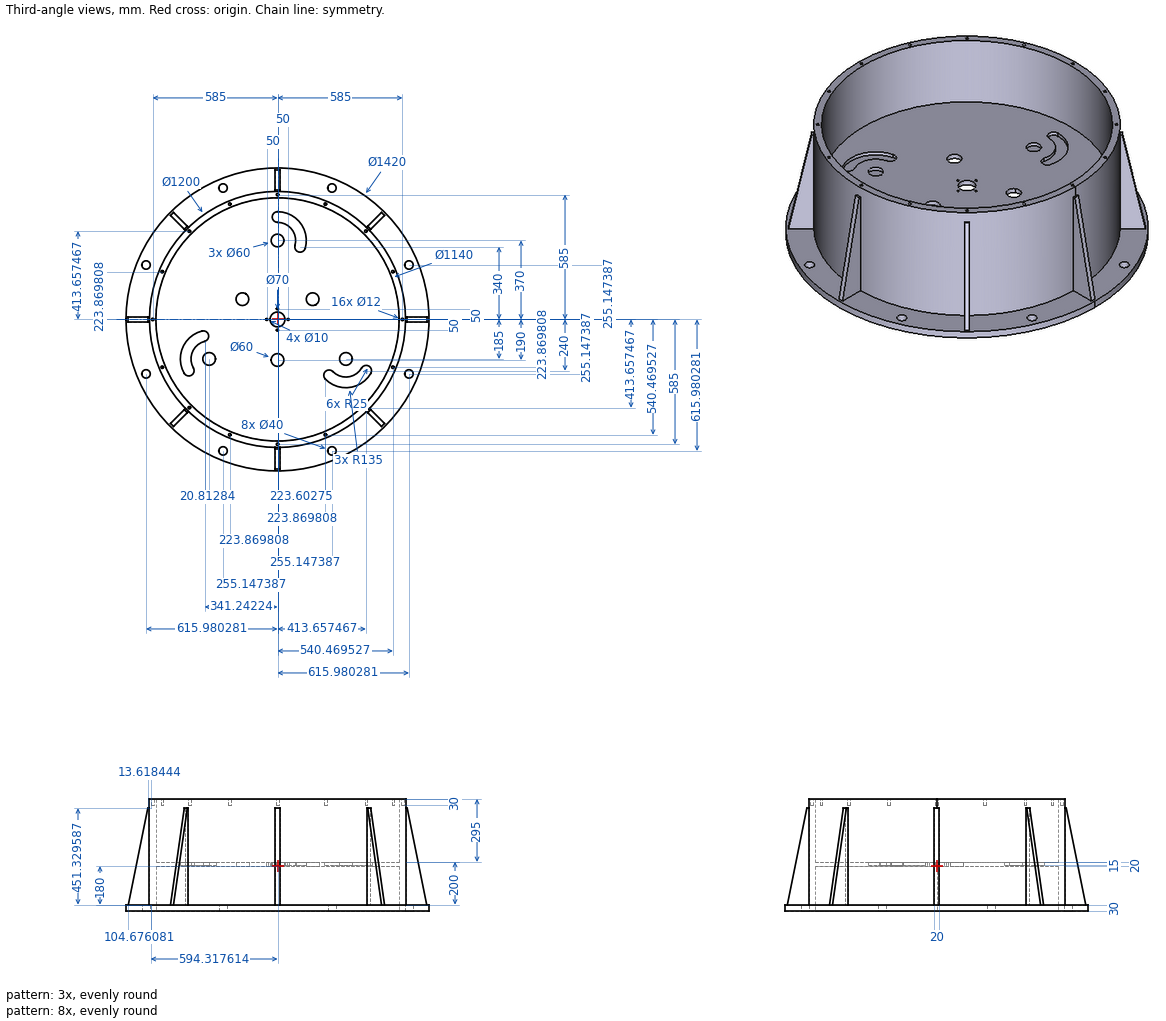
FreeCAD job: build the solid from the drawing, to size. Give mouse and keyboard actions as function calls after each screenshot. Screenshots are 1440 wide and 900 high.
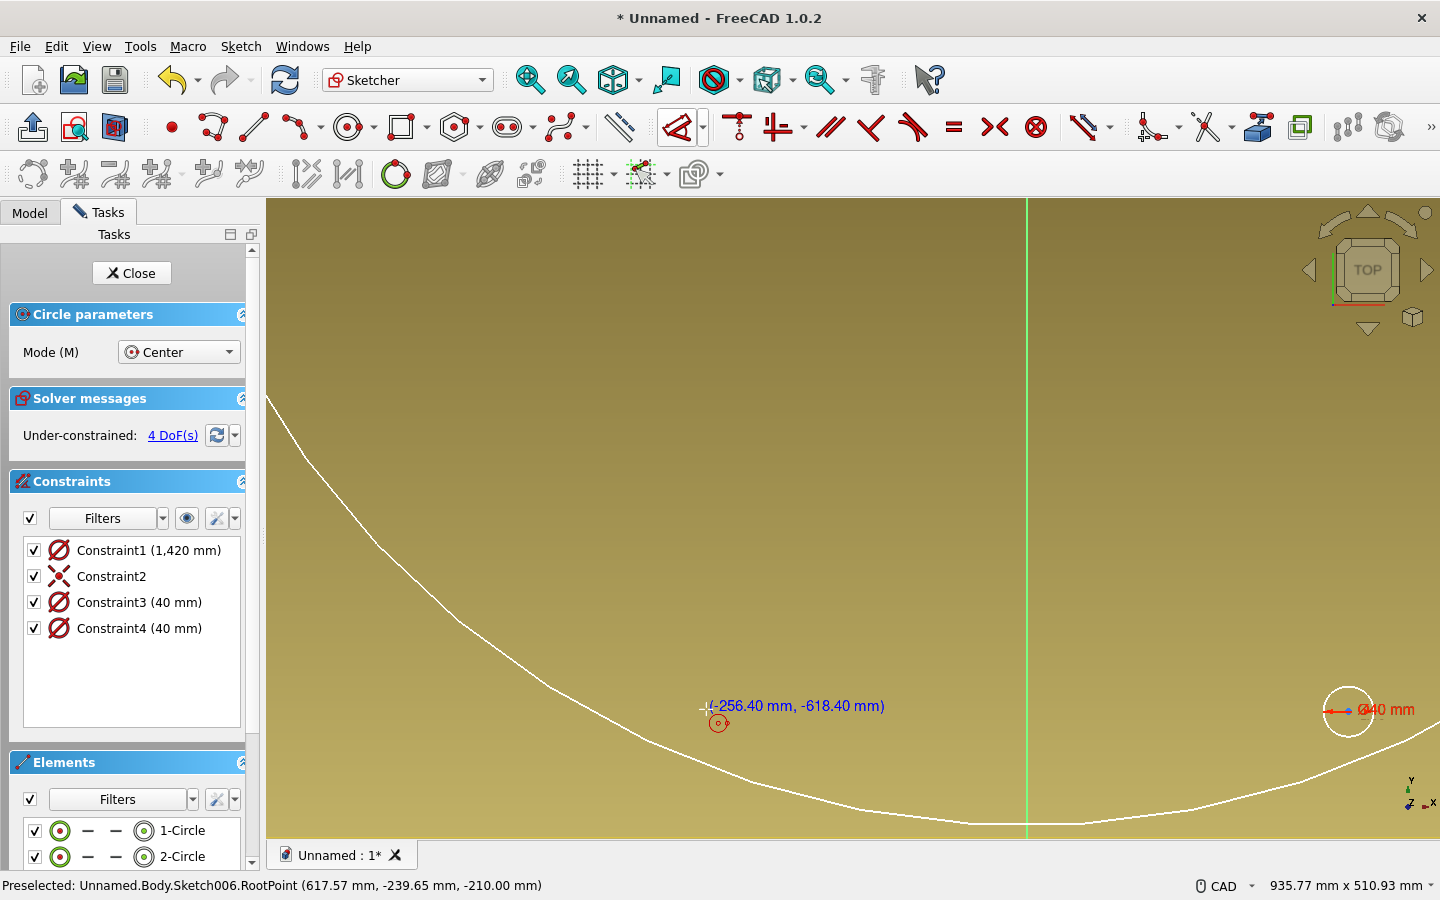
scroll(705, 710, down, 7)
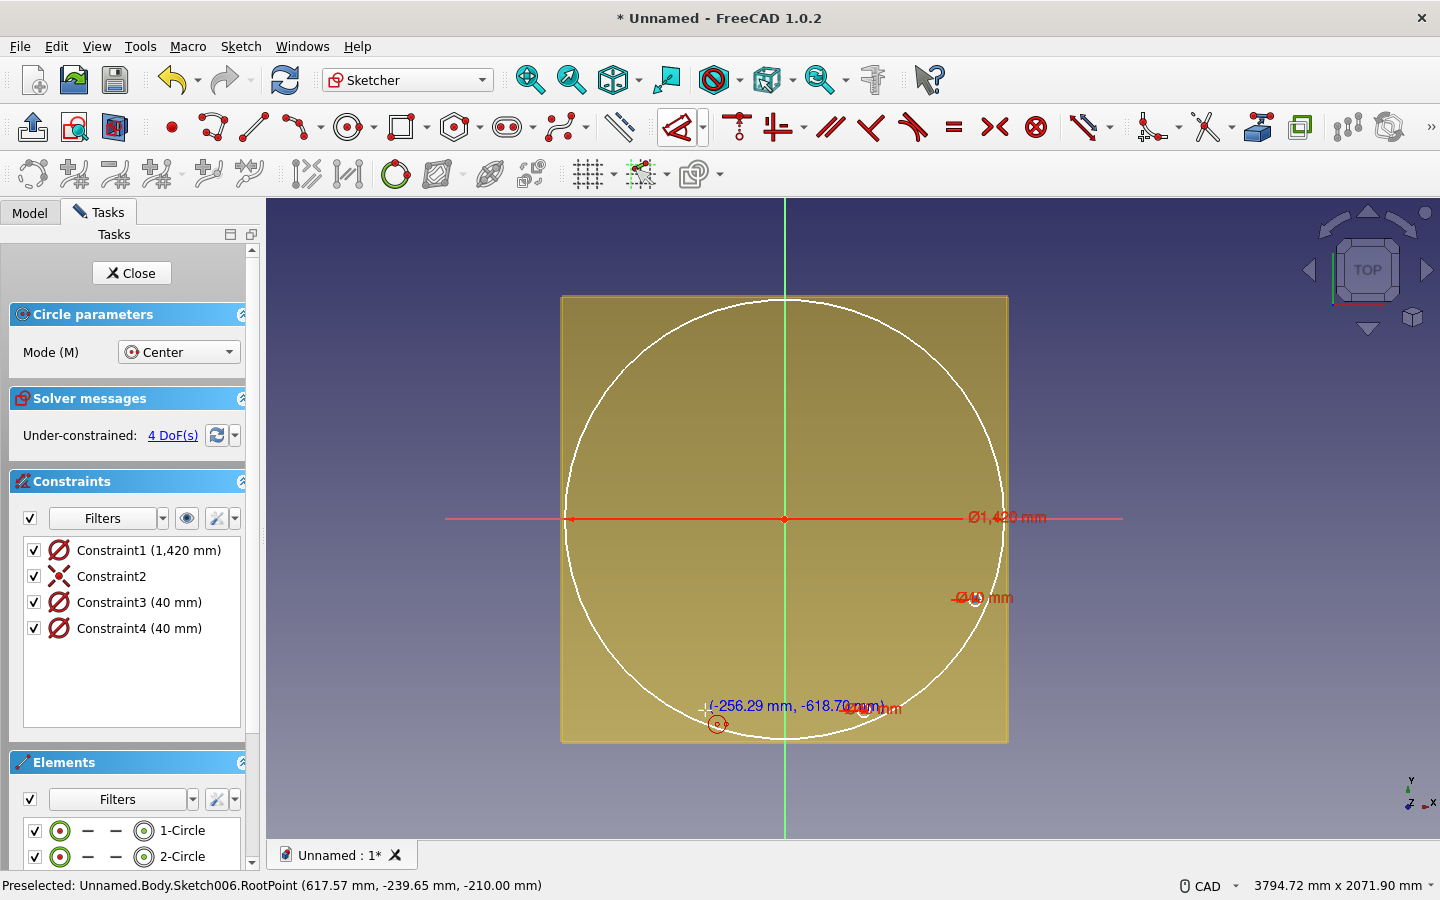
click(706, 710)
move(710, 706)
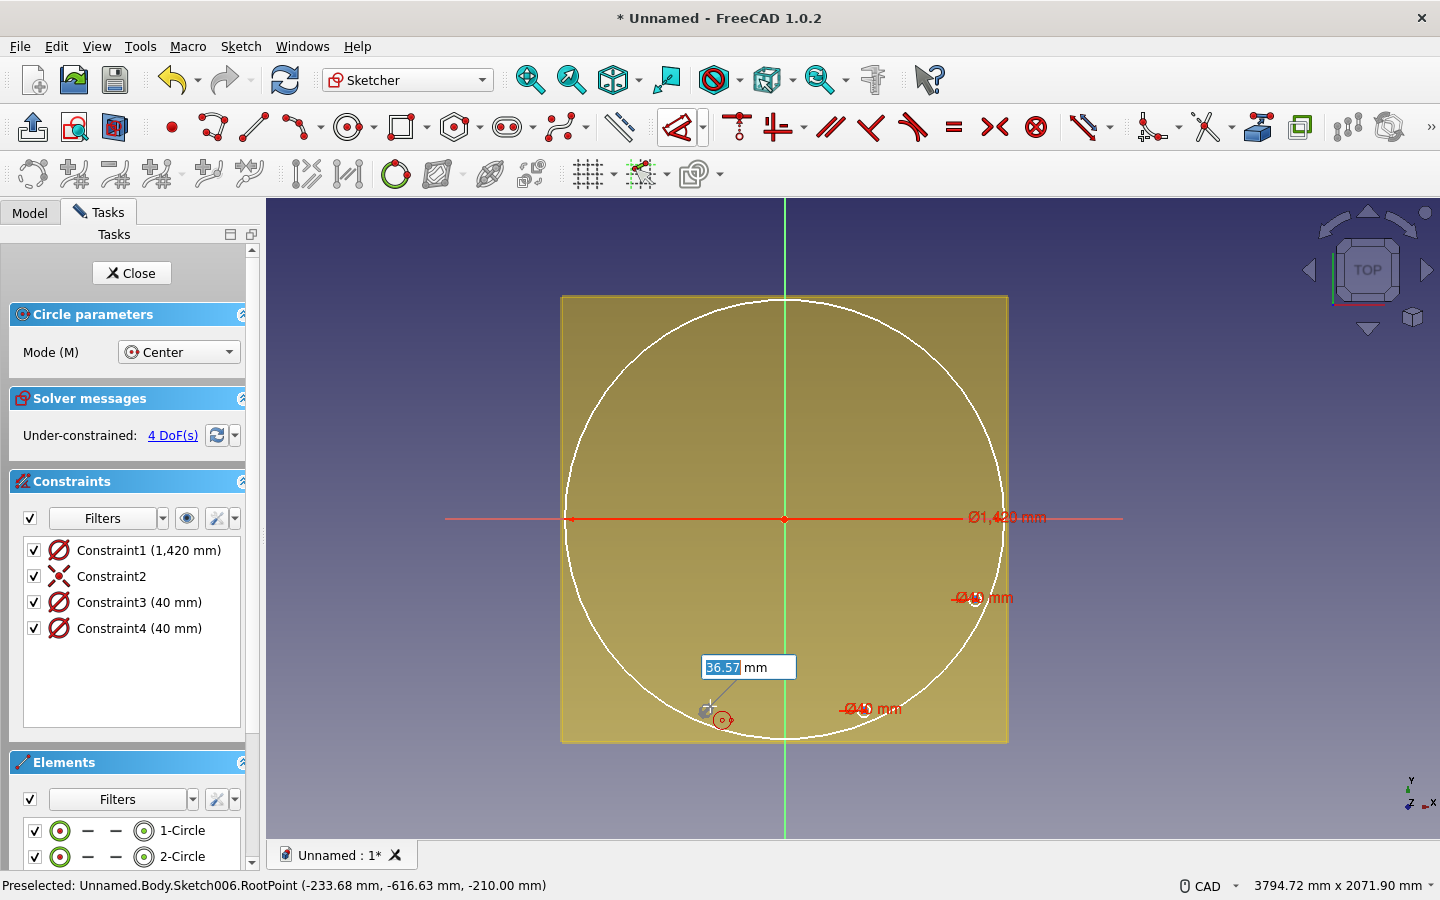
text(40)
key(Return)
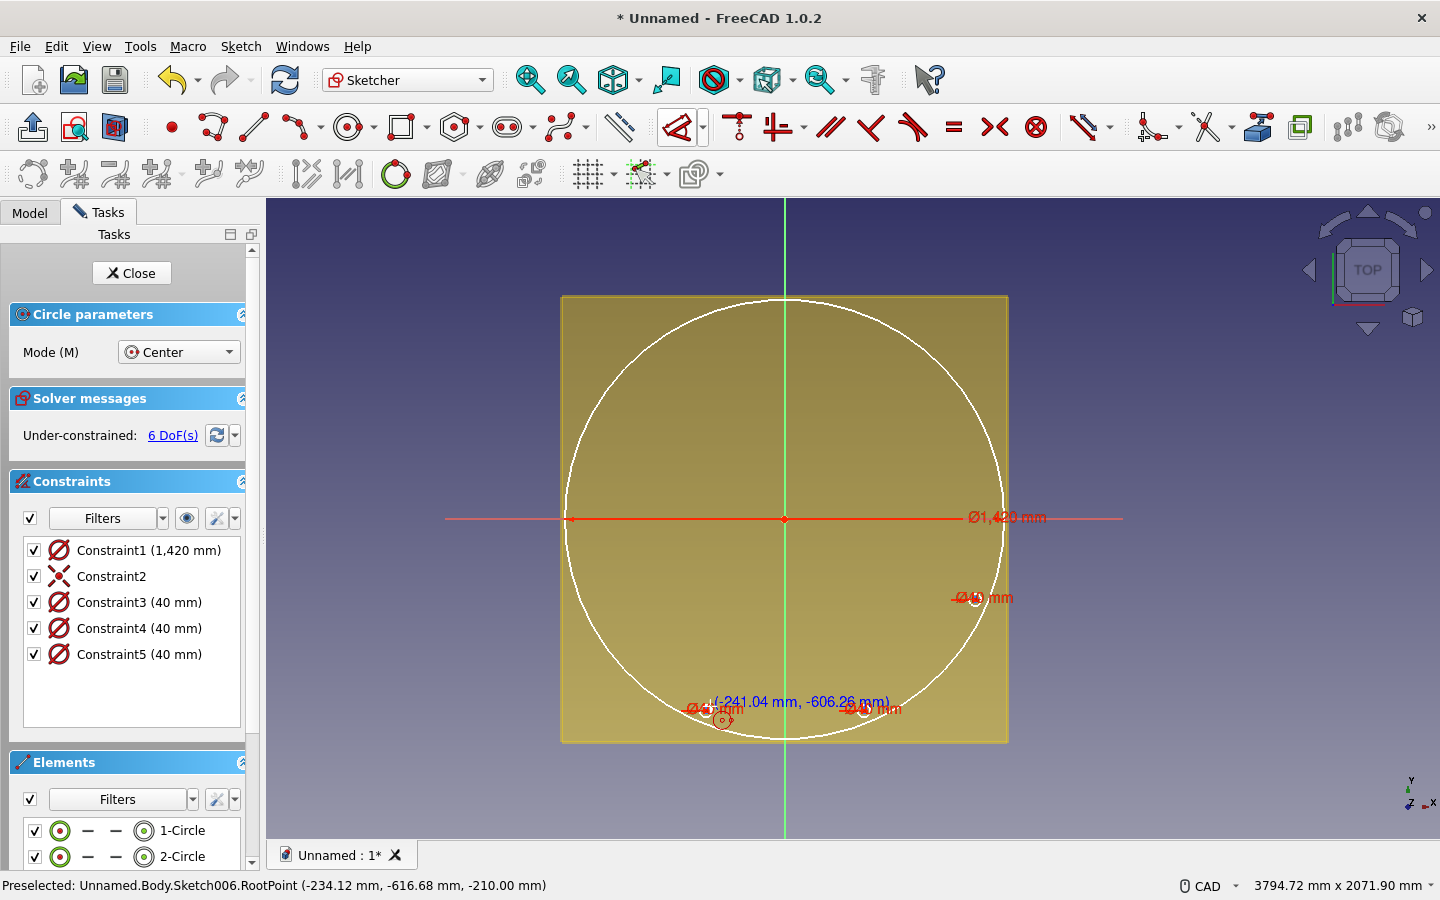
scroll(594, 598, up, 7)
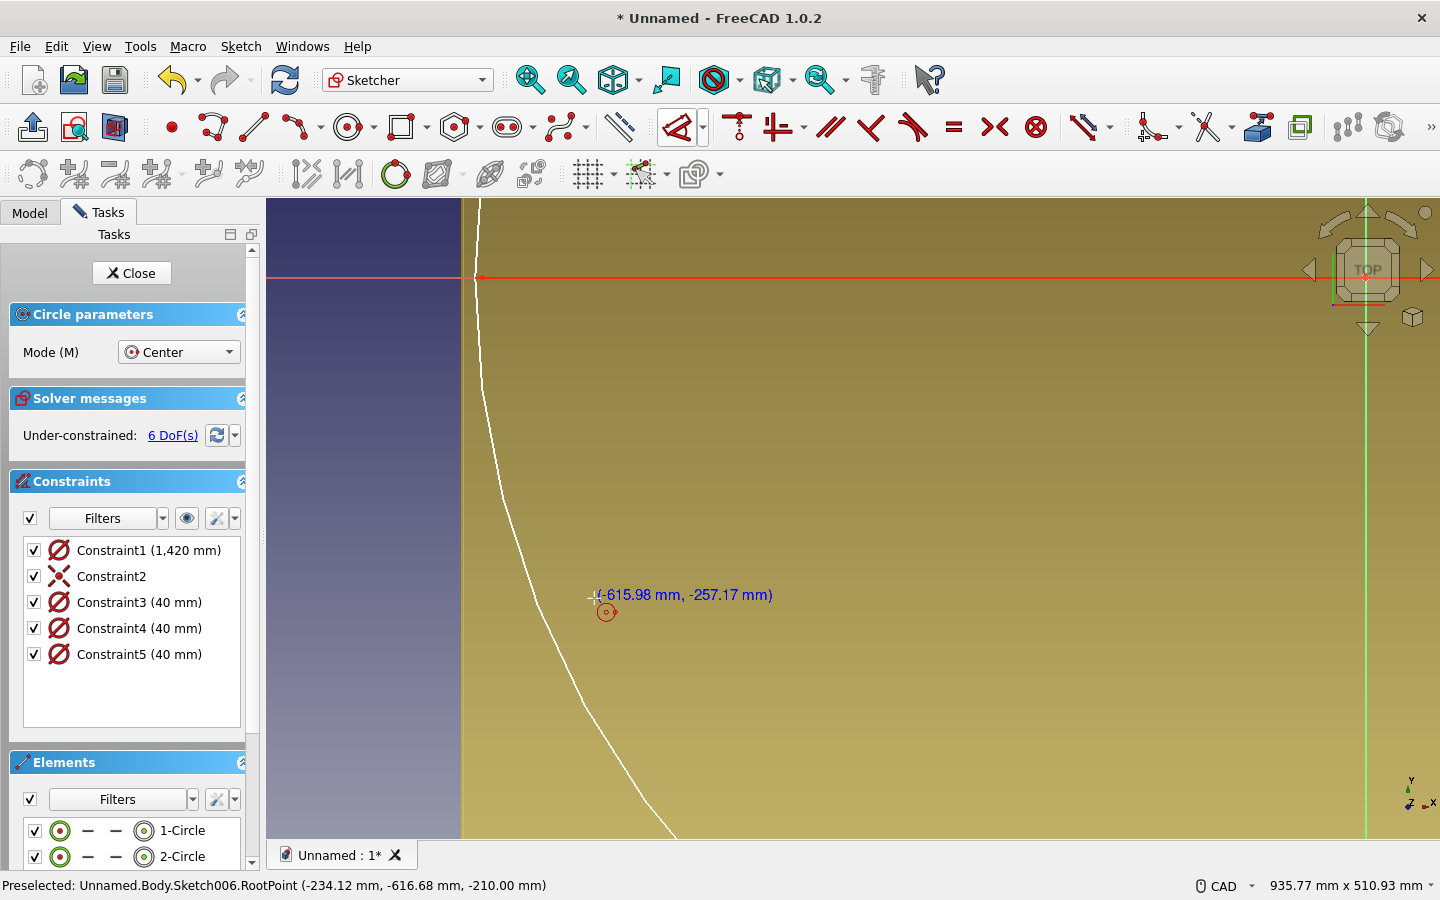
scroll(594, 597, down, 7)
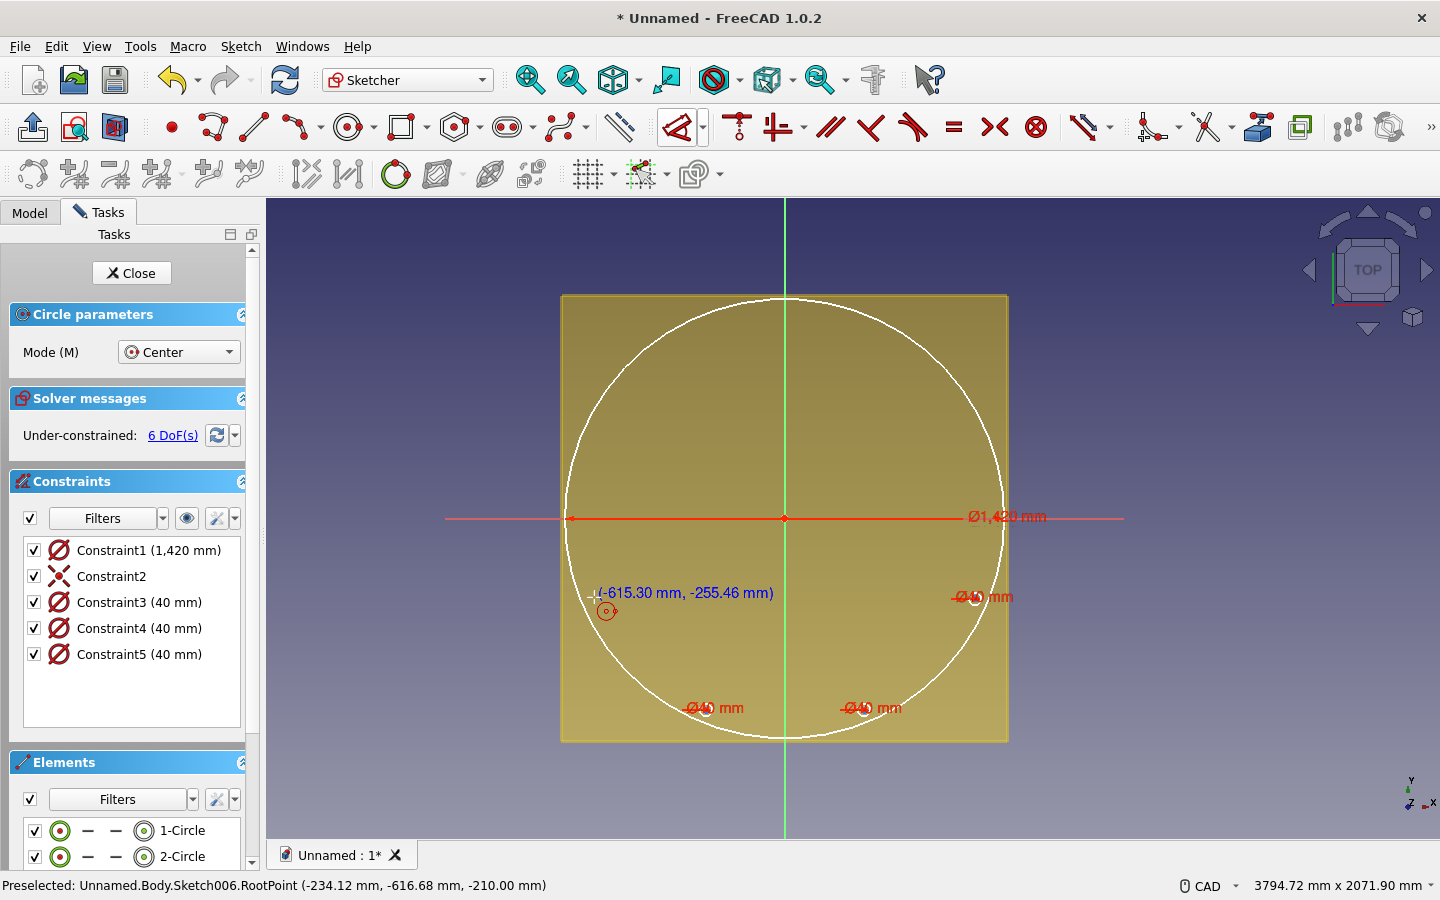
click(594, 598)
move(598, 593)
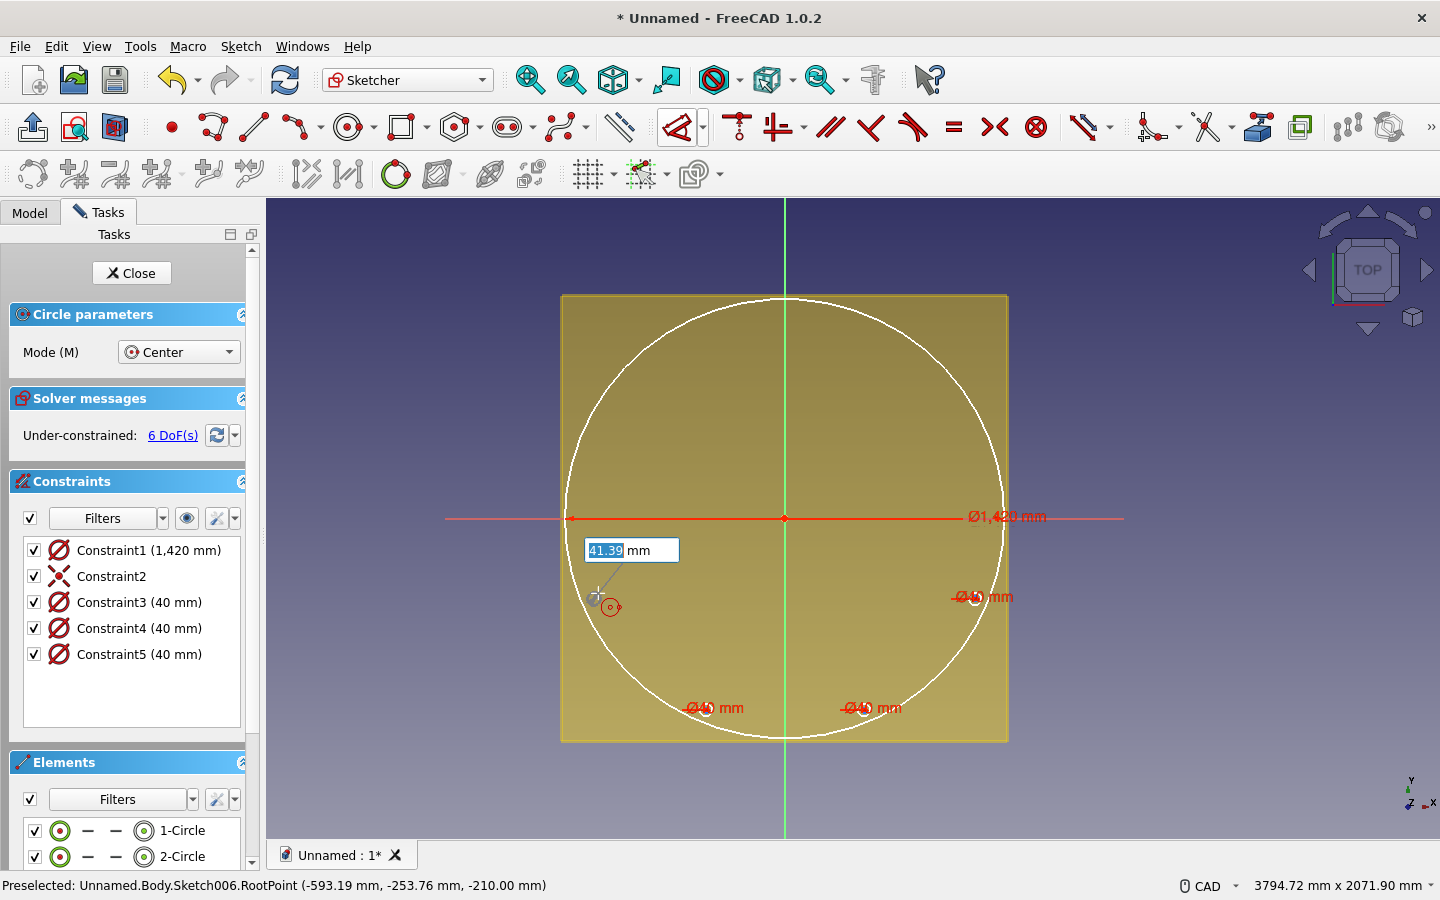
text(40)
key(Return)